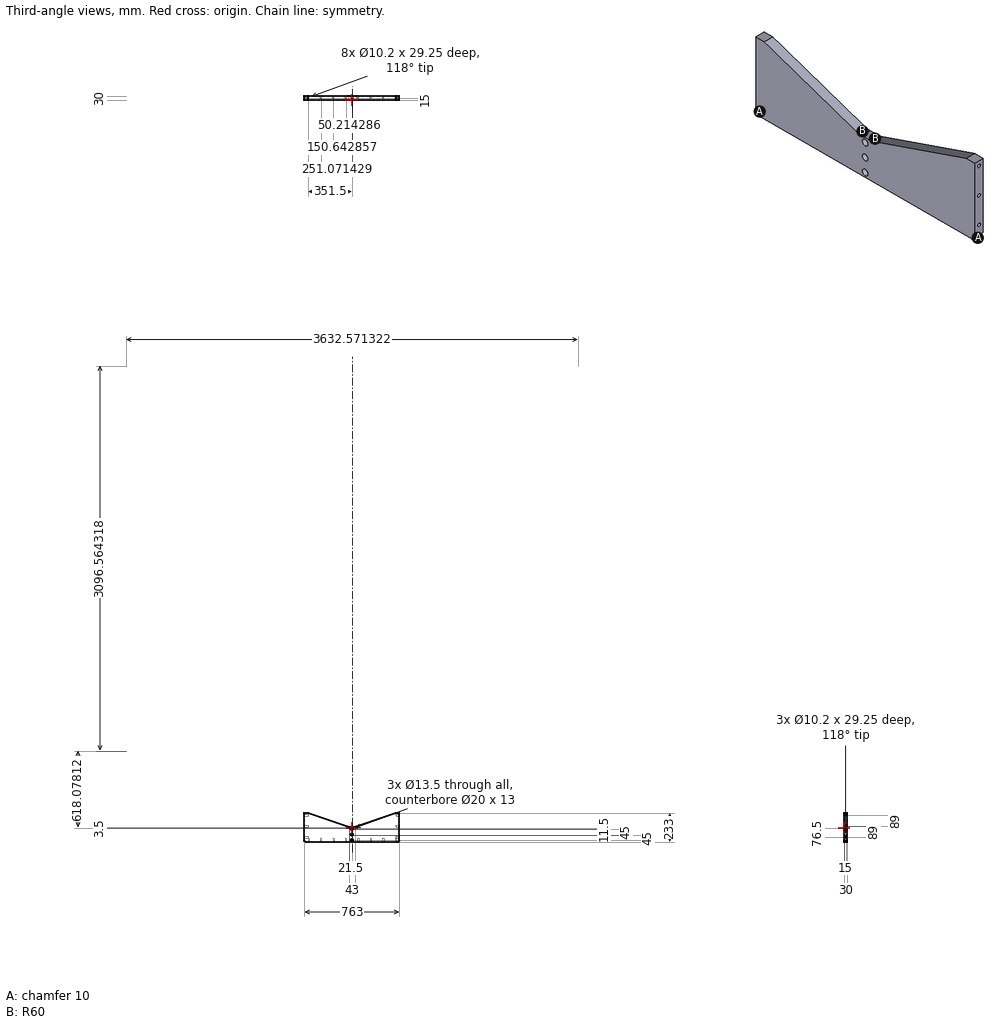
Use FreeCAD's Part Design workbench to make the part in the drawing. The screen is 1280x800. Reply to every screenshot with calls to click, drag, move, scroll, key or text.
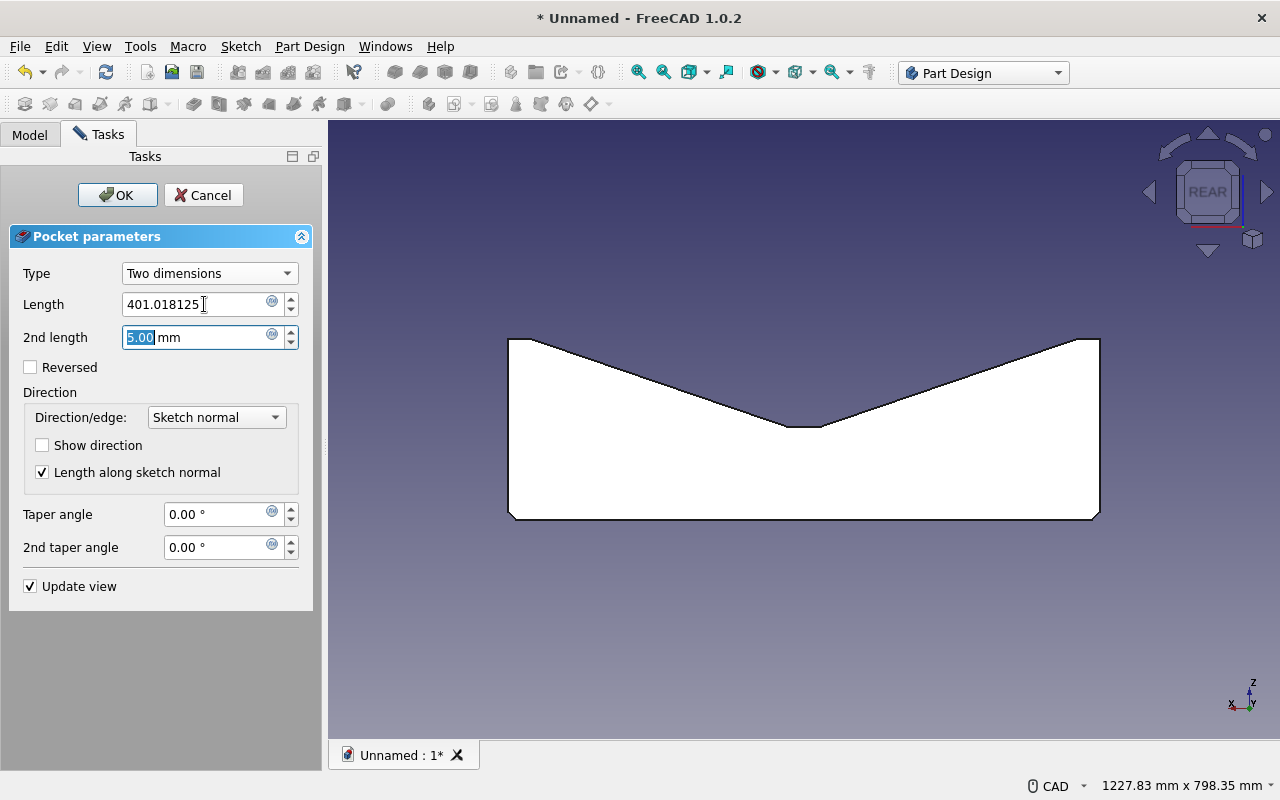
text(30)
key(Tab)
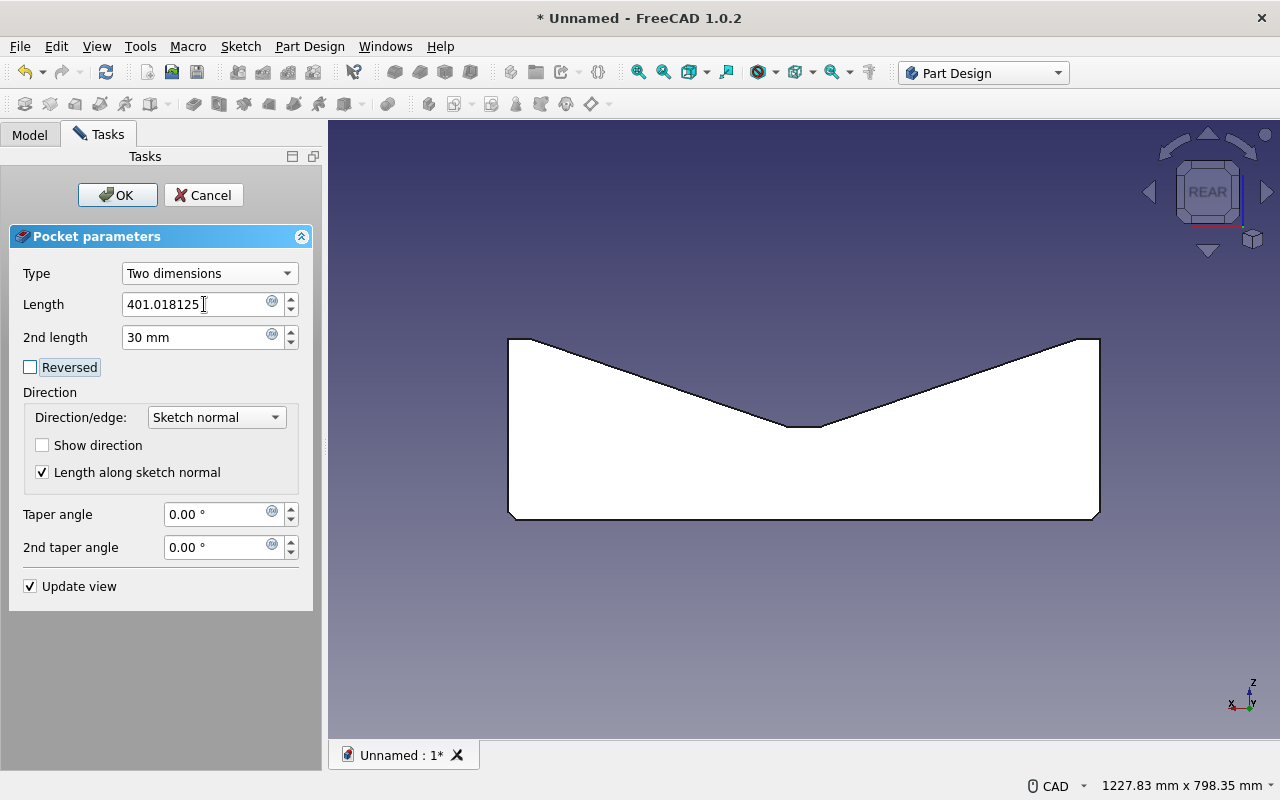
click(31, 367)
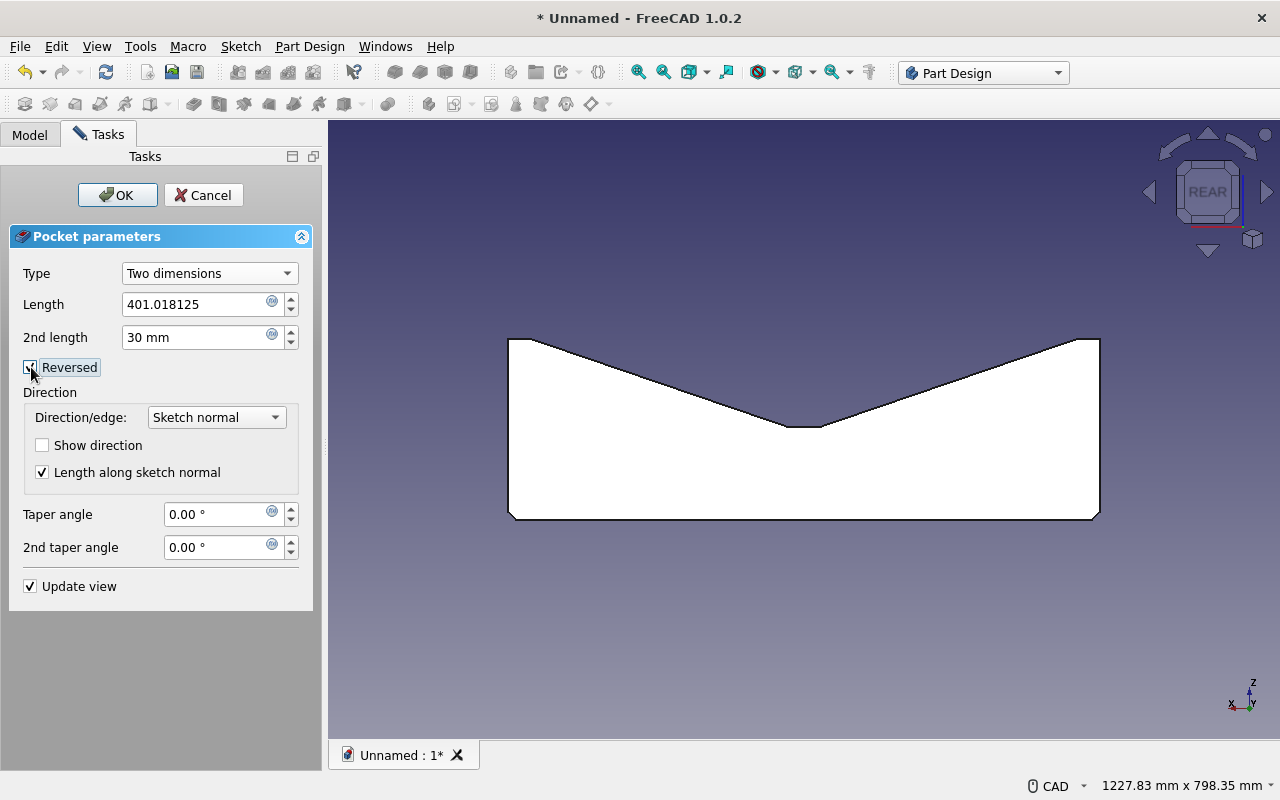
click(118, 195)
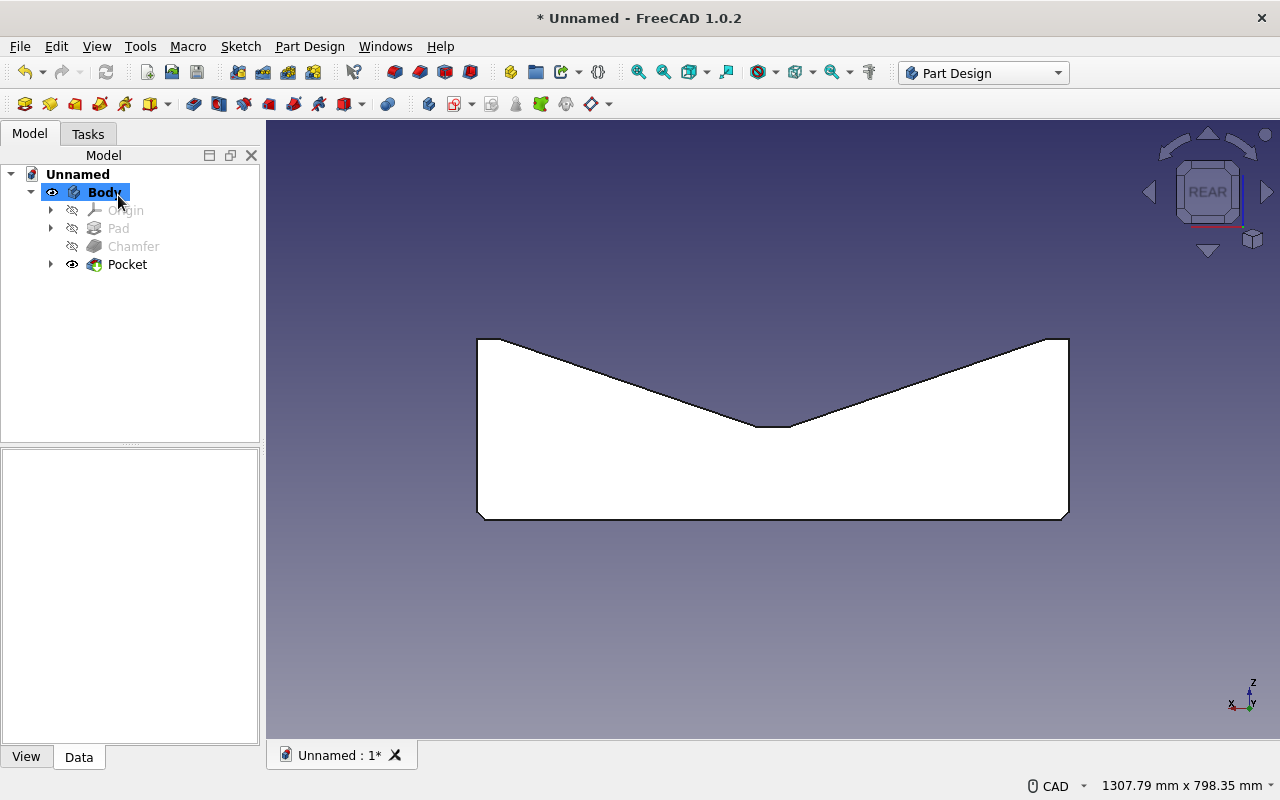
key(0)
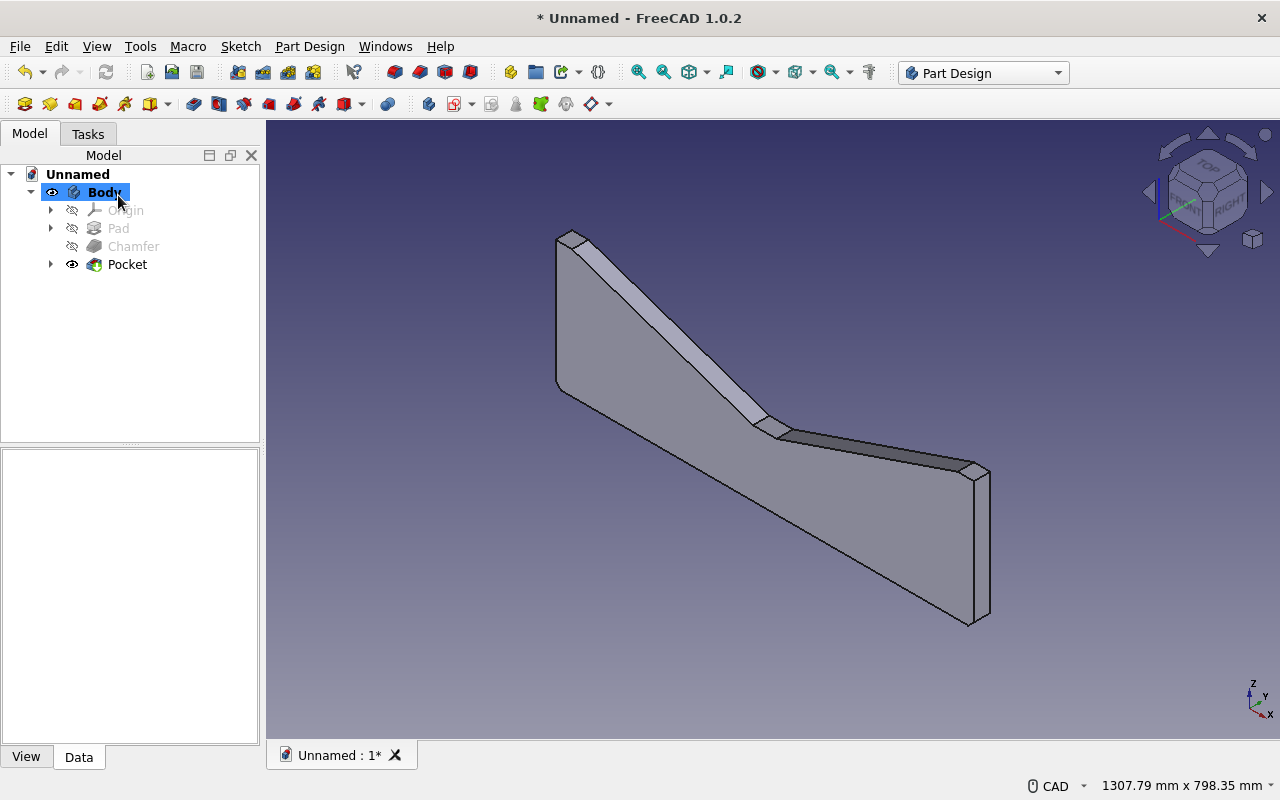
key(2)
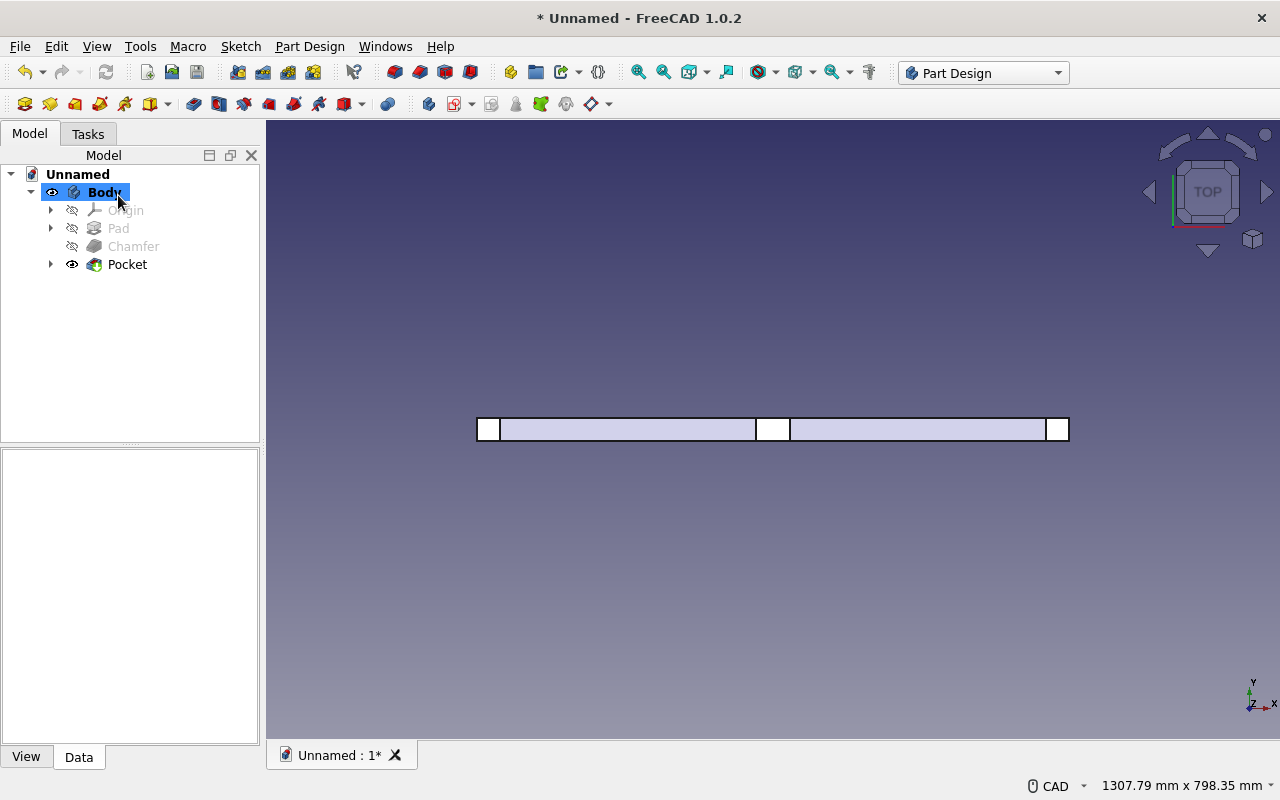
key(1)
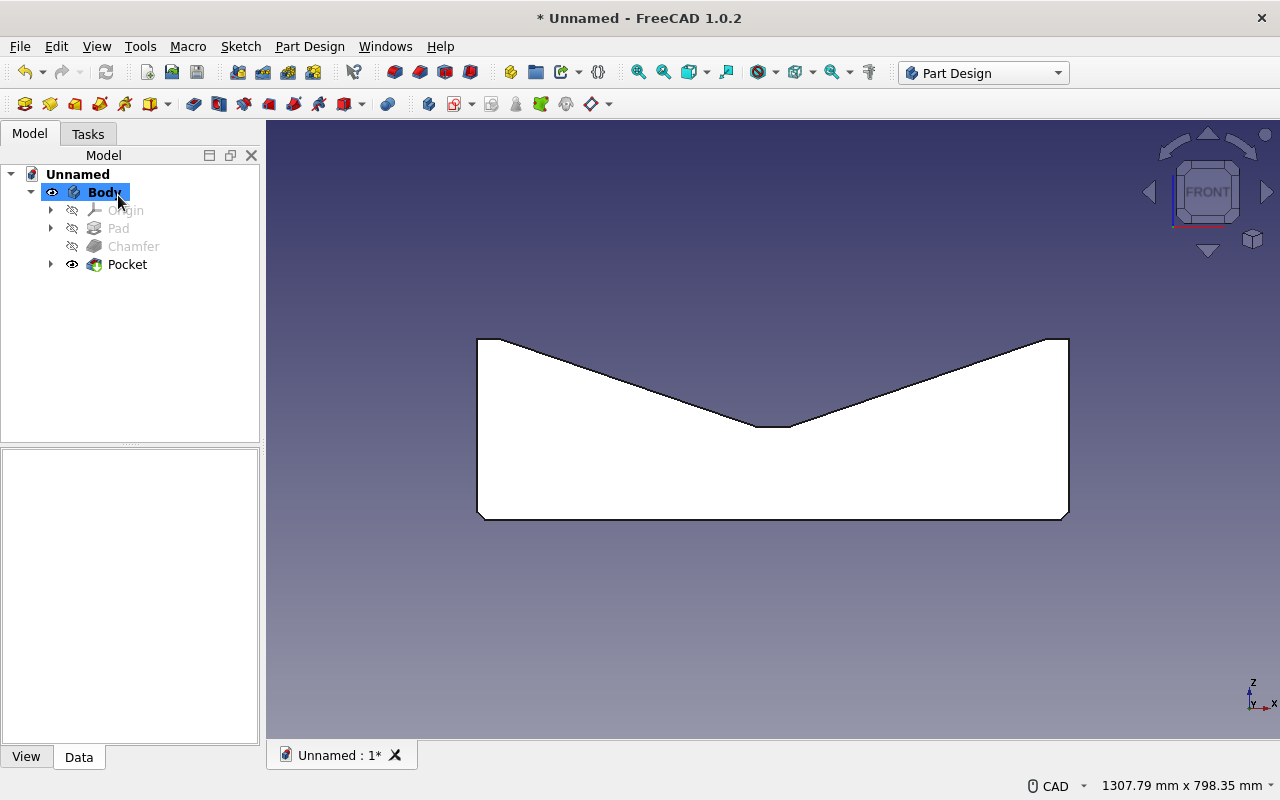
key(3)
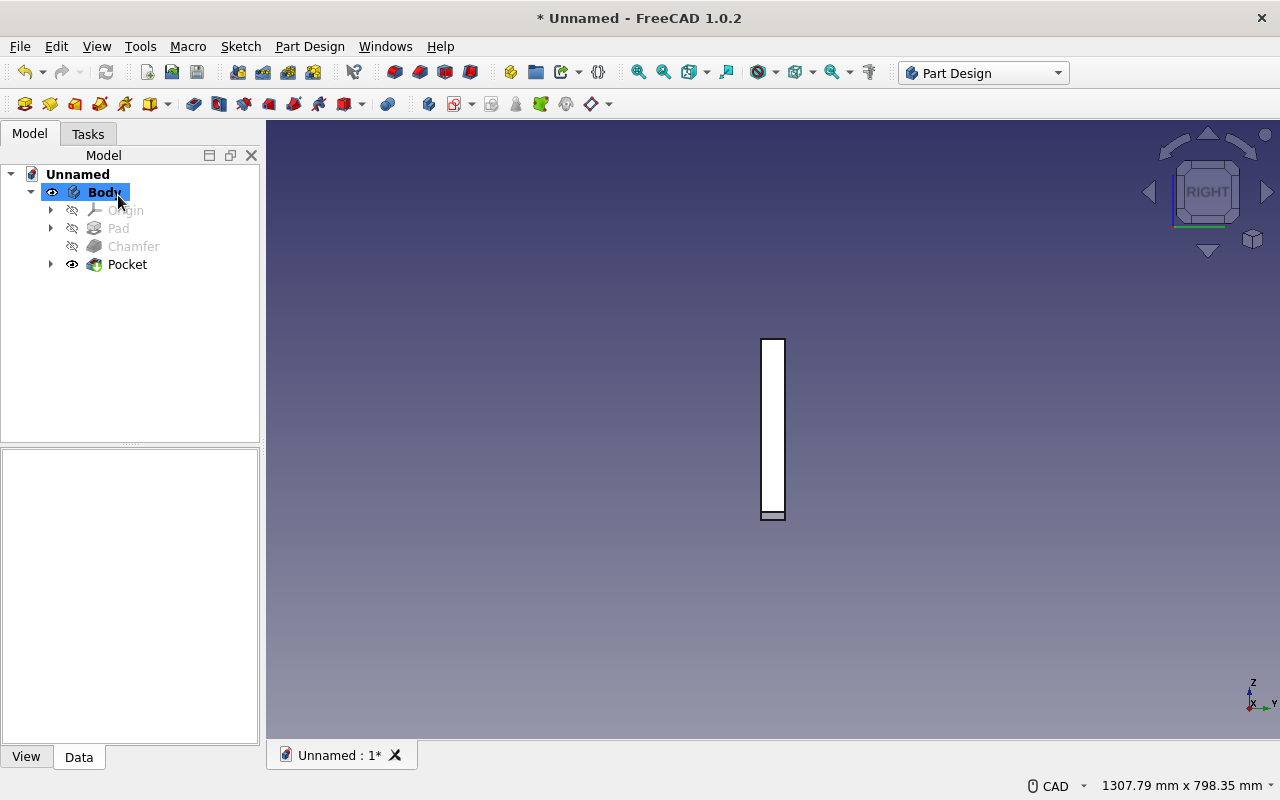
key(v)
key(f)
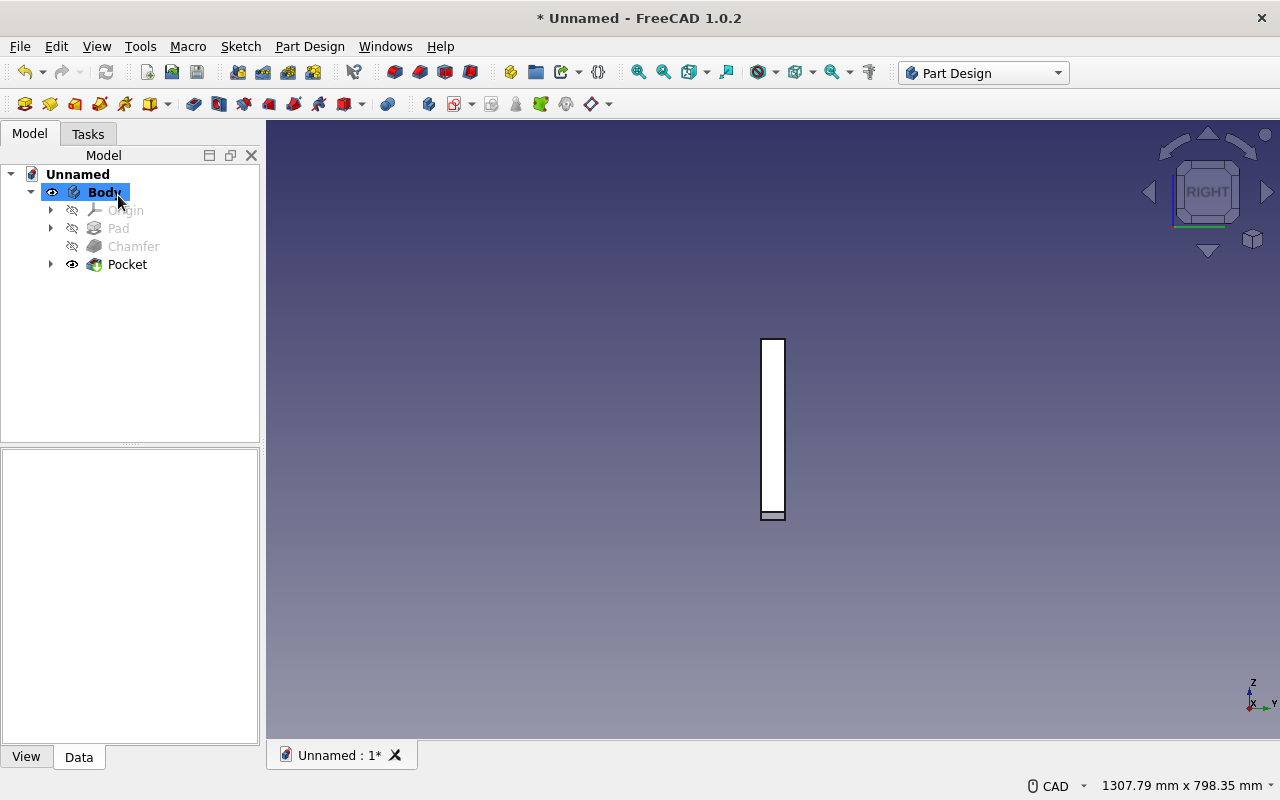
key(5)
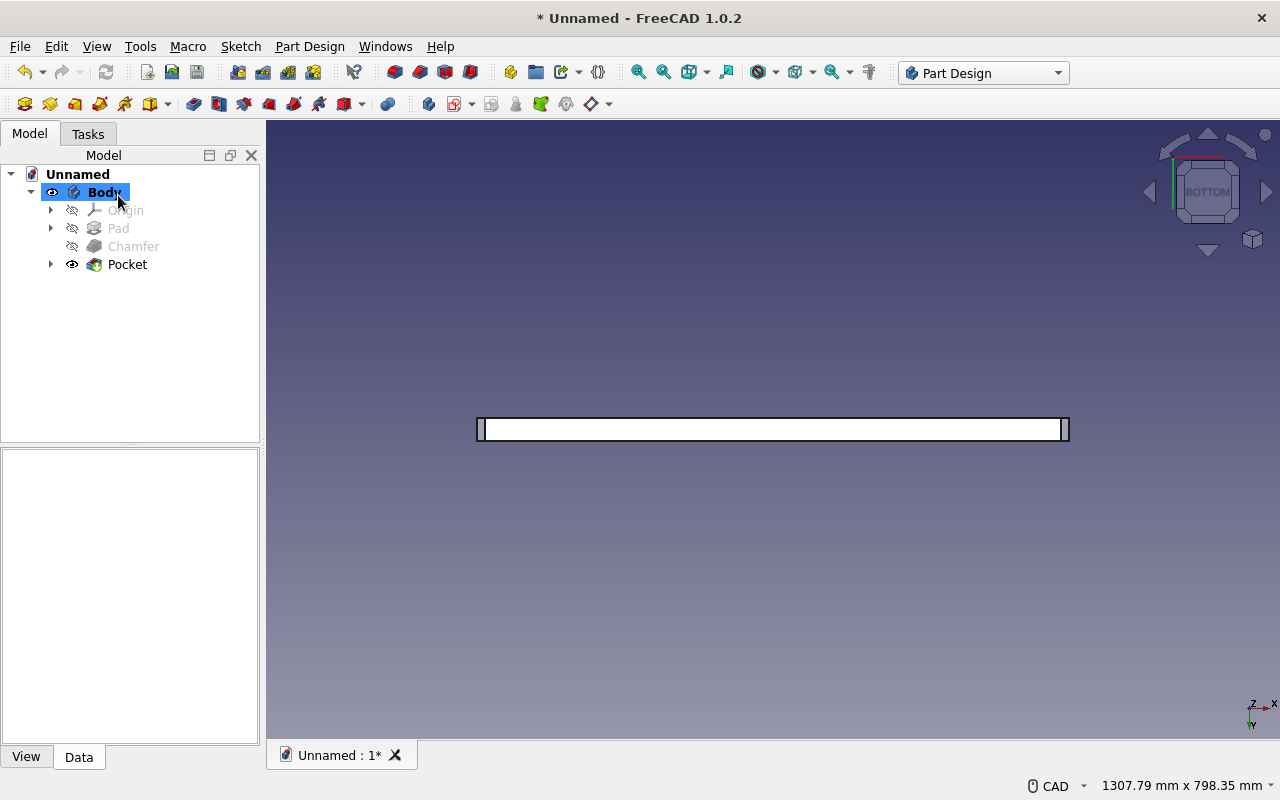
key(4)